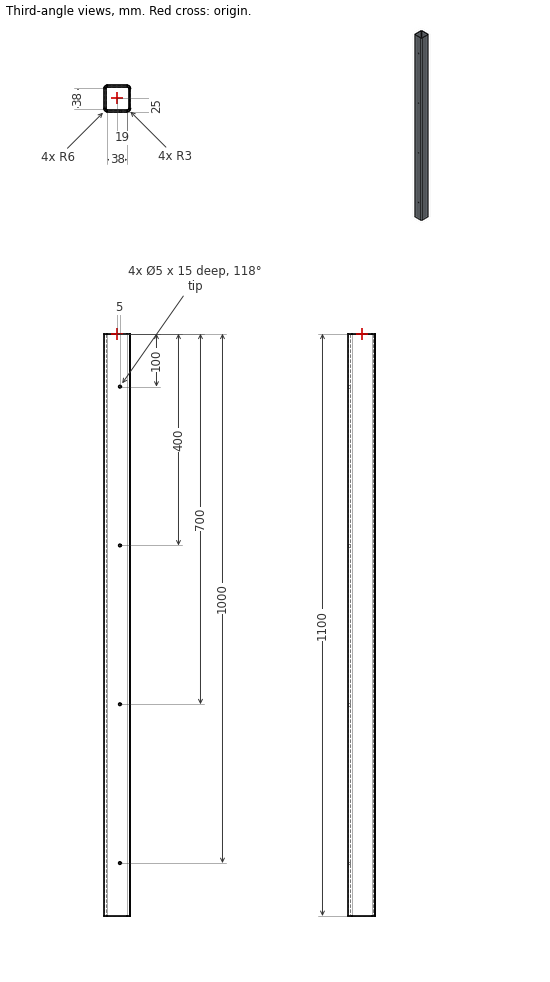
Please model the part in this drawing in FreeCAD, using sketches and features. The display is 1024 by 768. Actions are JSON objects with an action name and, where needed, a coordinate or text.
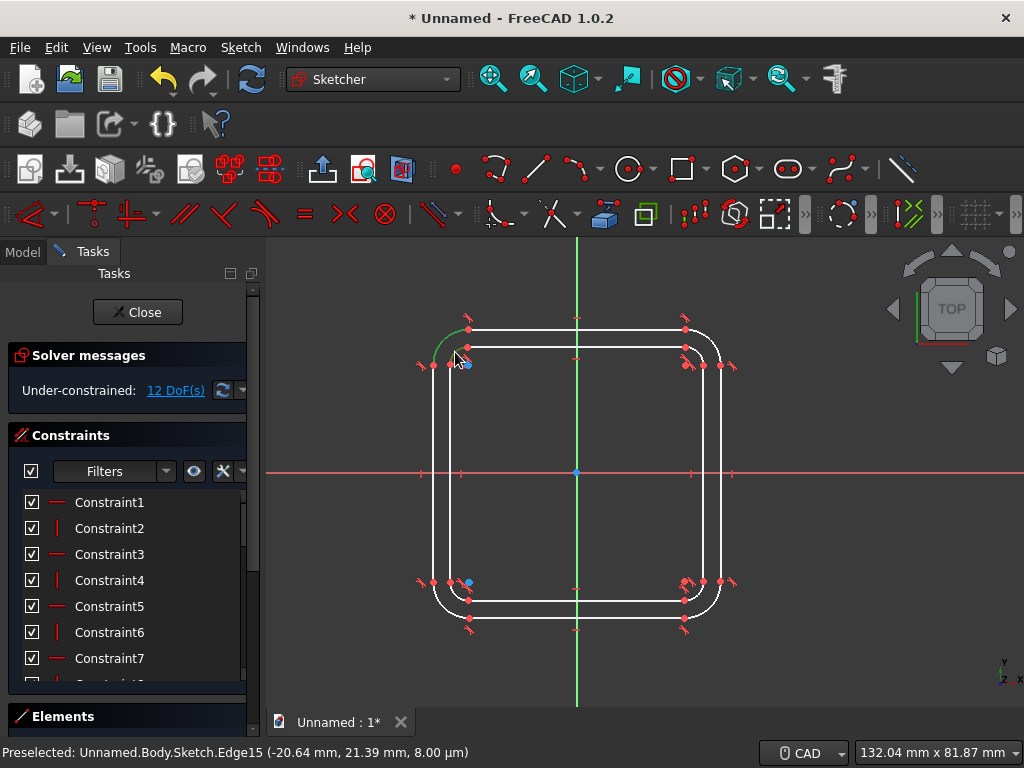
{"action": "left_click", "coordinate": [92, 214]}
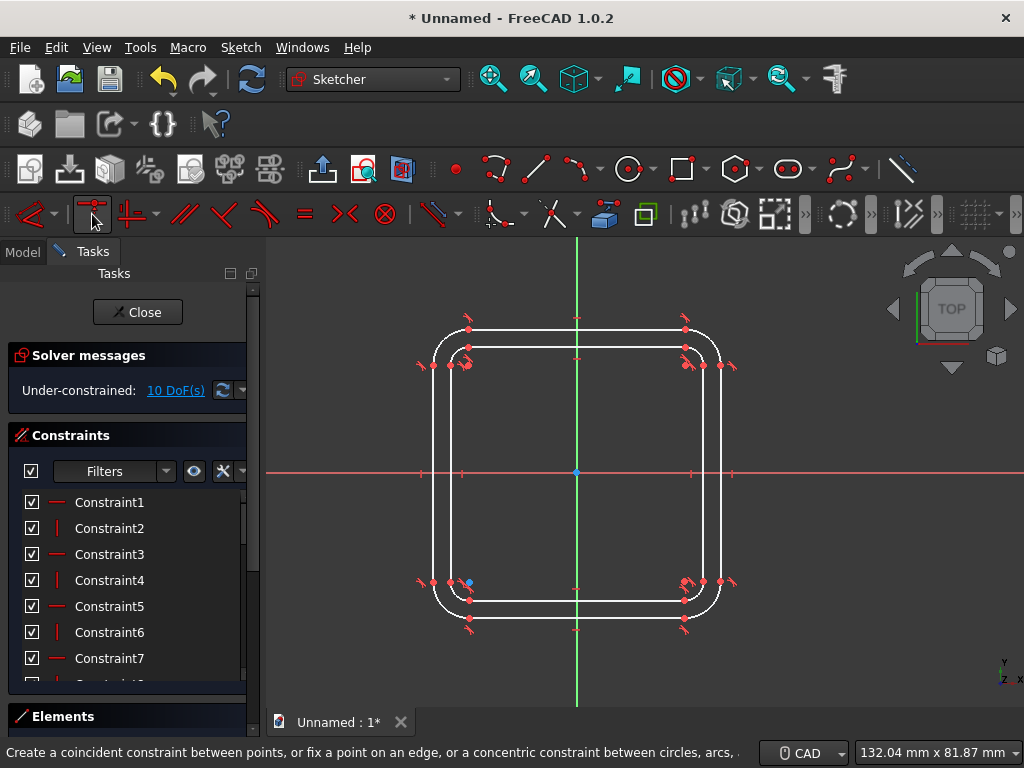
{"action": "left_click", "coordinate": [437, 599]}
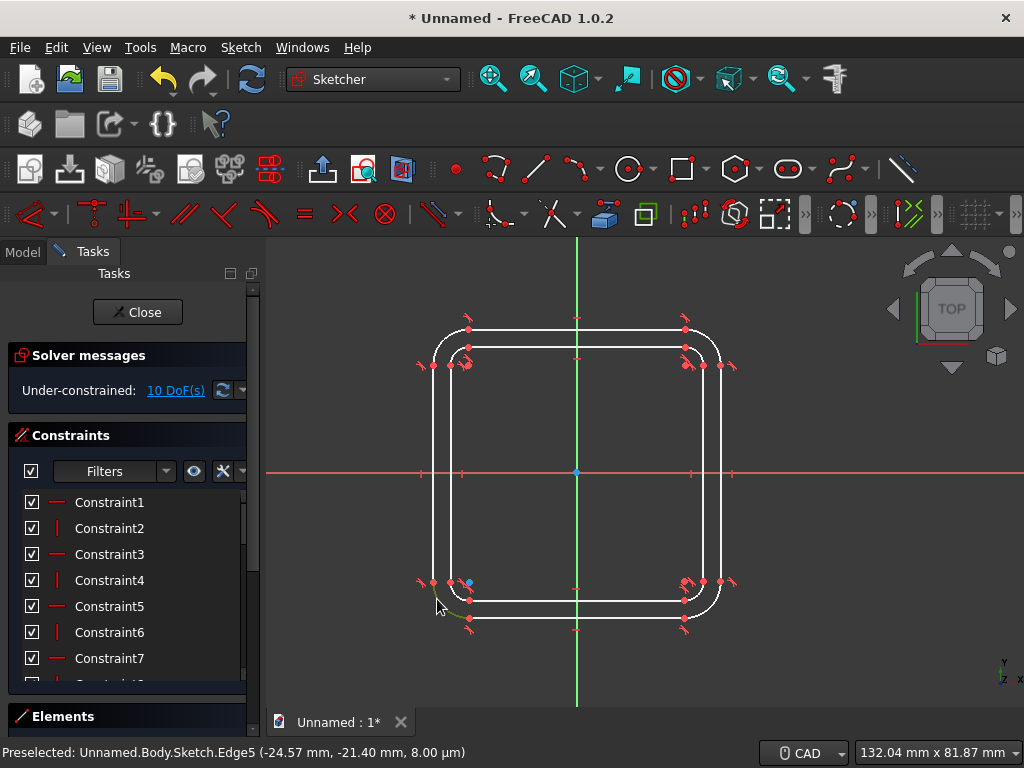
{"action": "left_click", "coordinate": [453, 334]}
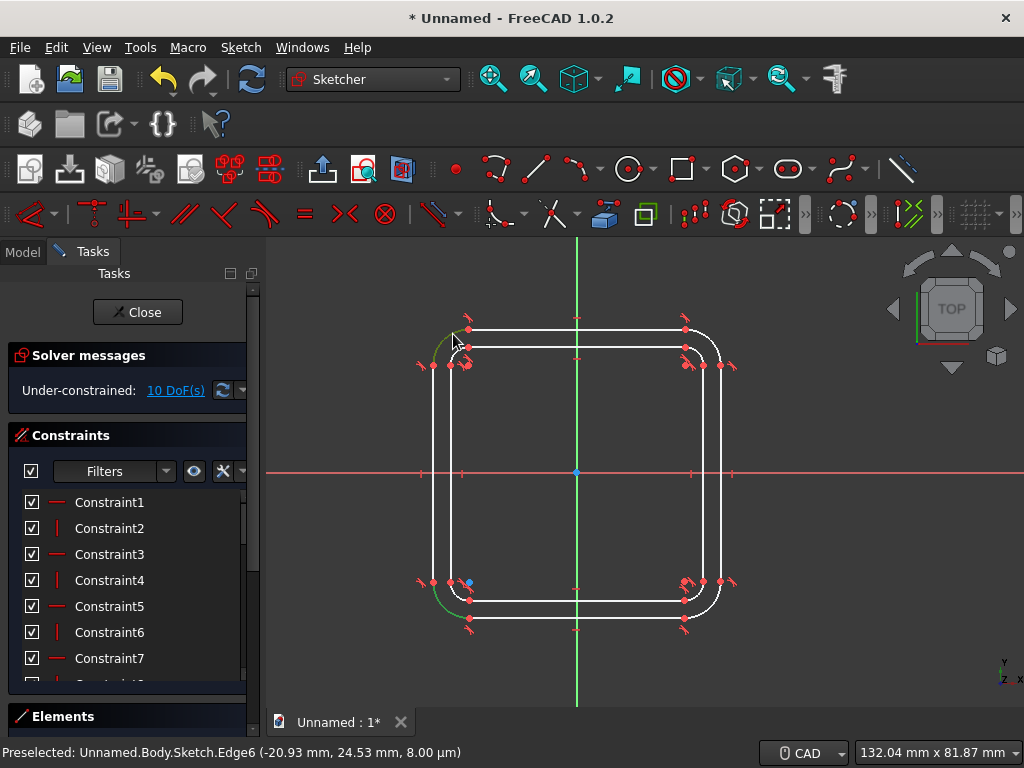
{"action": "left_click", "coordinate": [717, 349]}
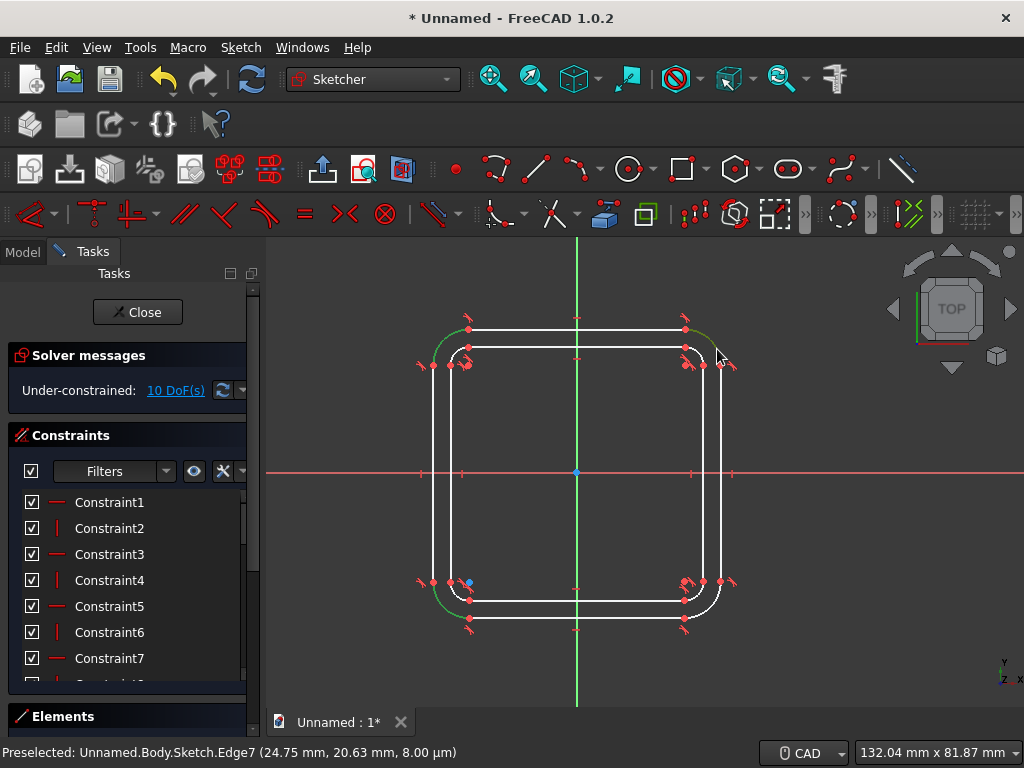
{"action": "left_click", "coordinate": [701, 614]}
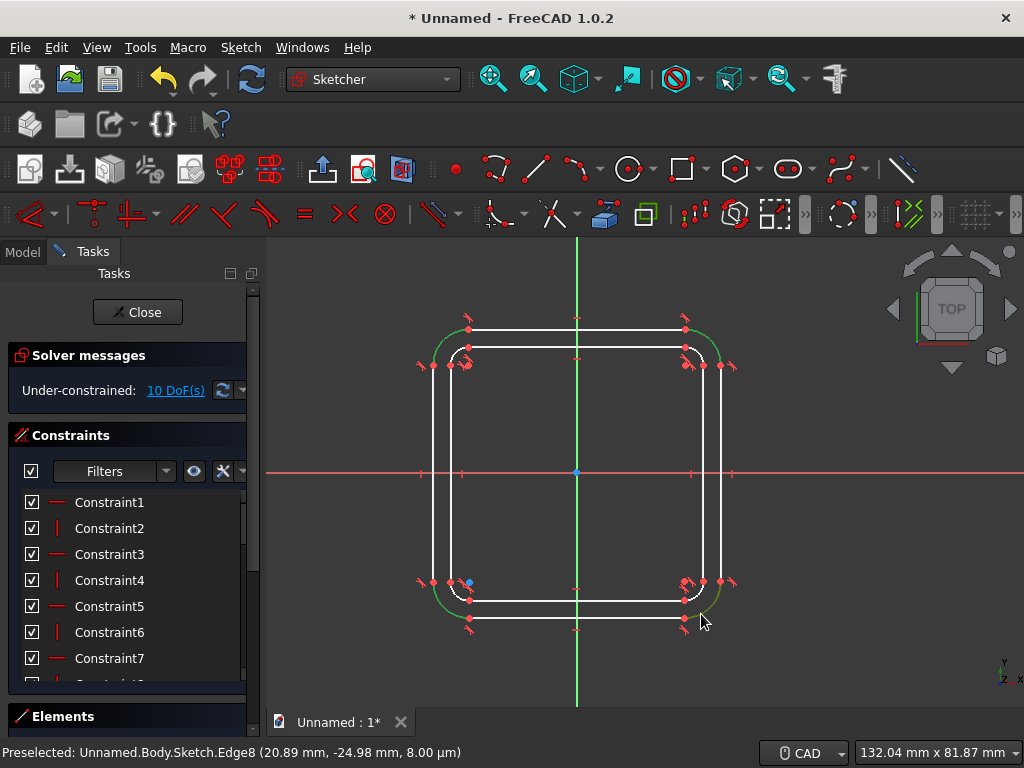
{"action": "key", "text": "e"}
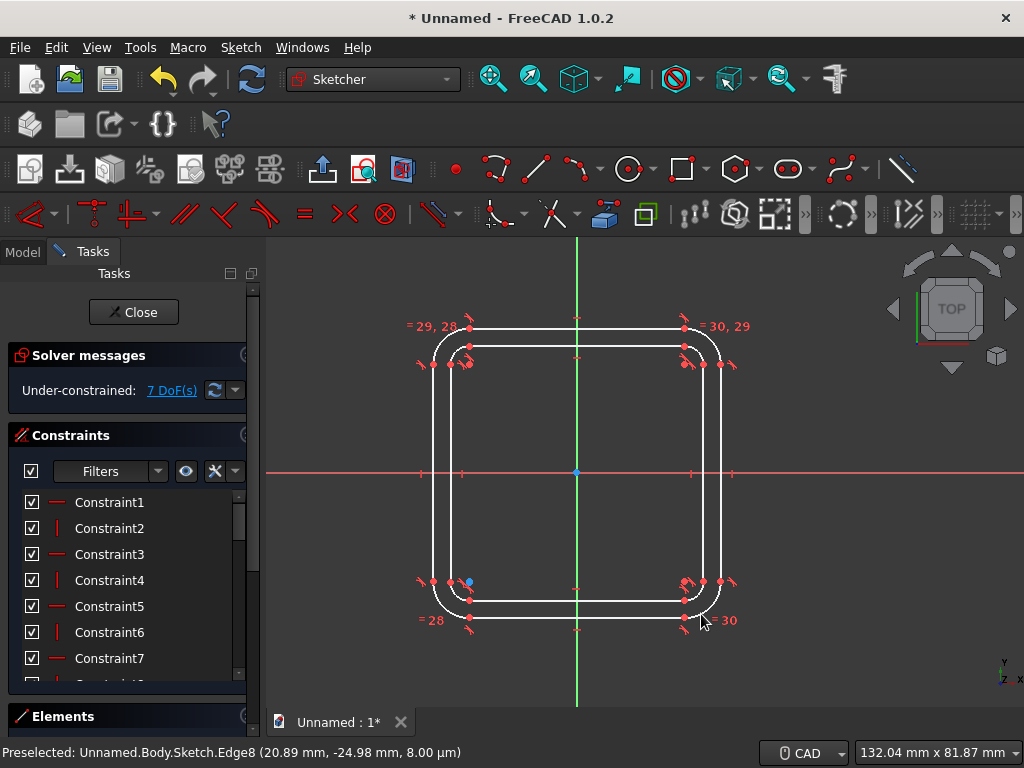
{"action": "left_click", "coordinate": [698, 595]}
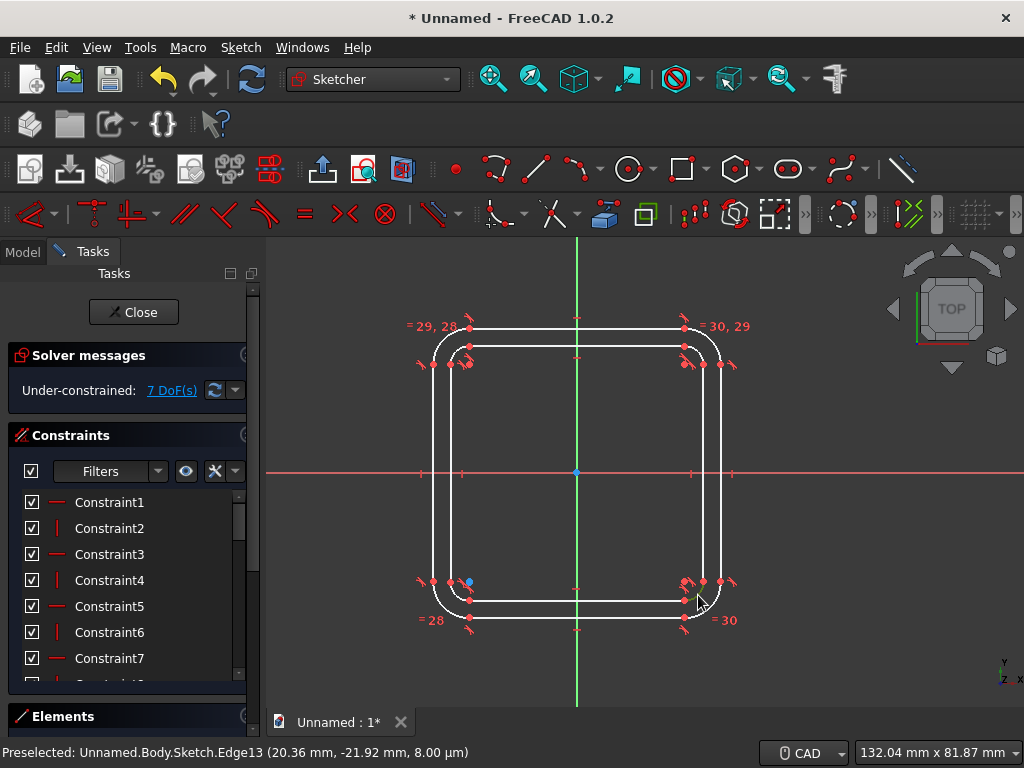
{"action": "left_click", "coordinate": [456, 595]}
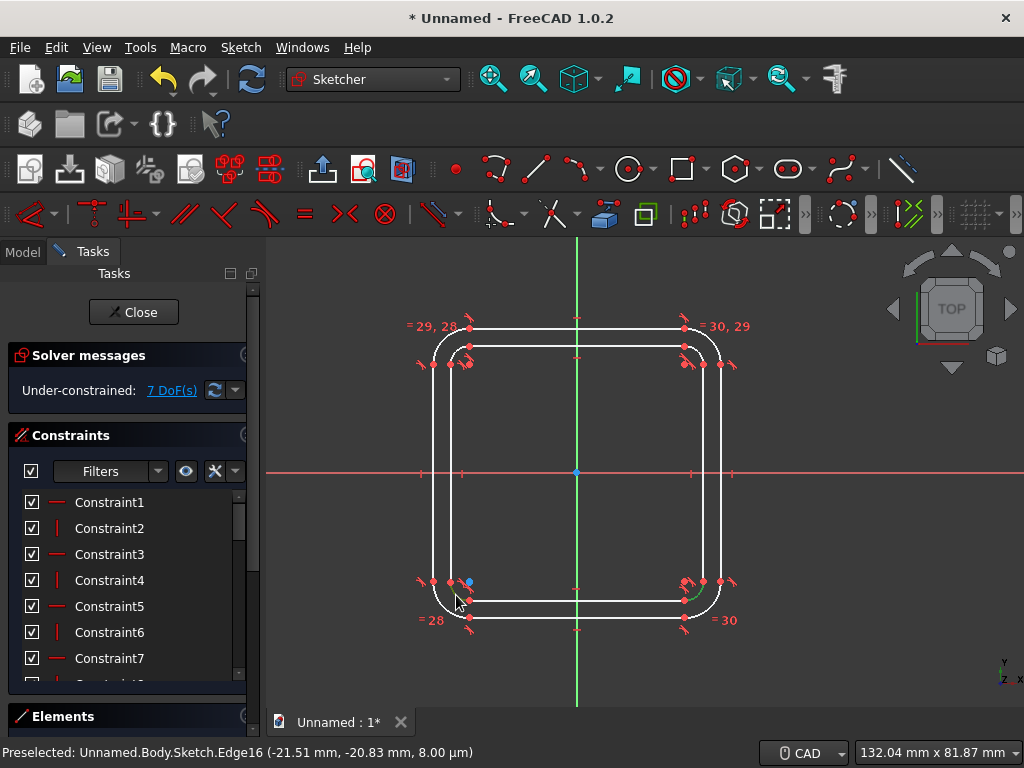
{"action": "left_click", "coordinate": [306, 214]}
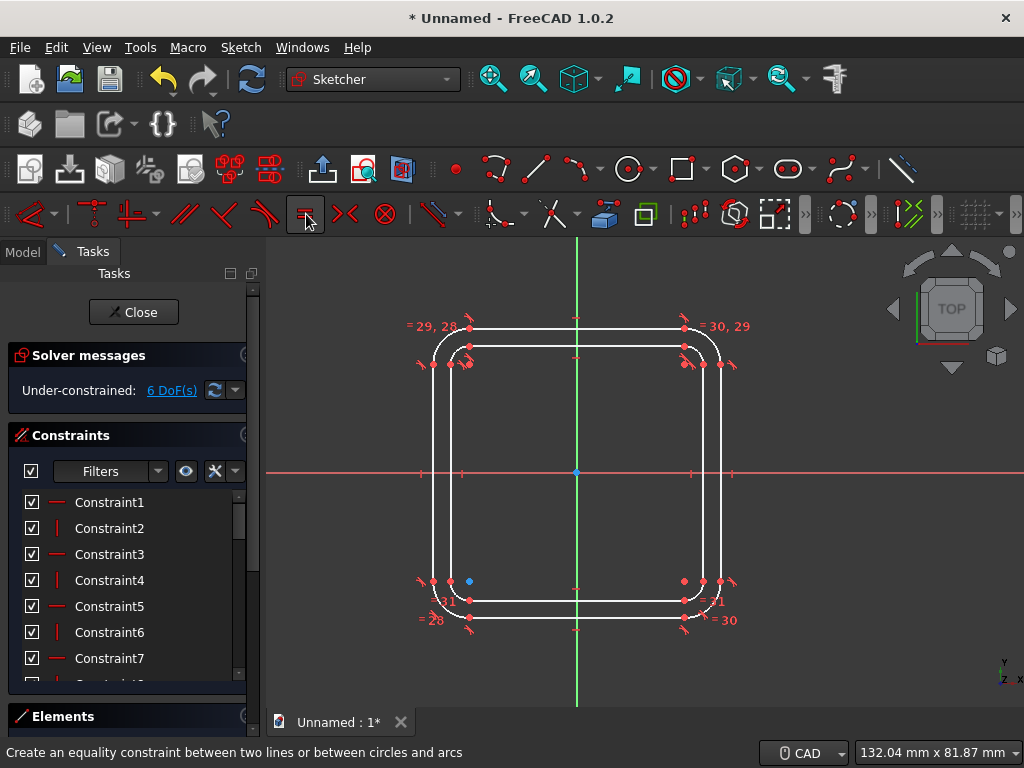
{"action": "left_click", "coordinate": [458, 616]}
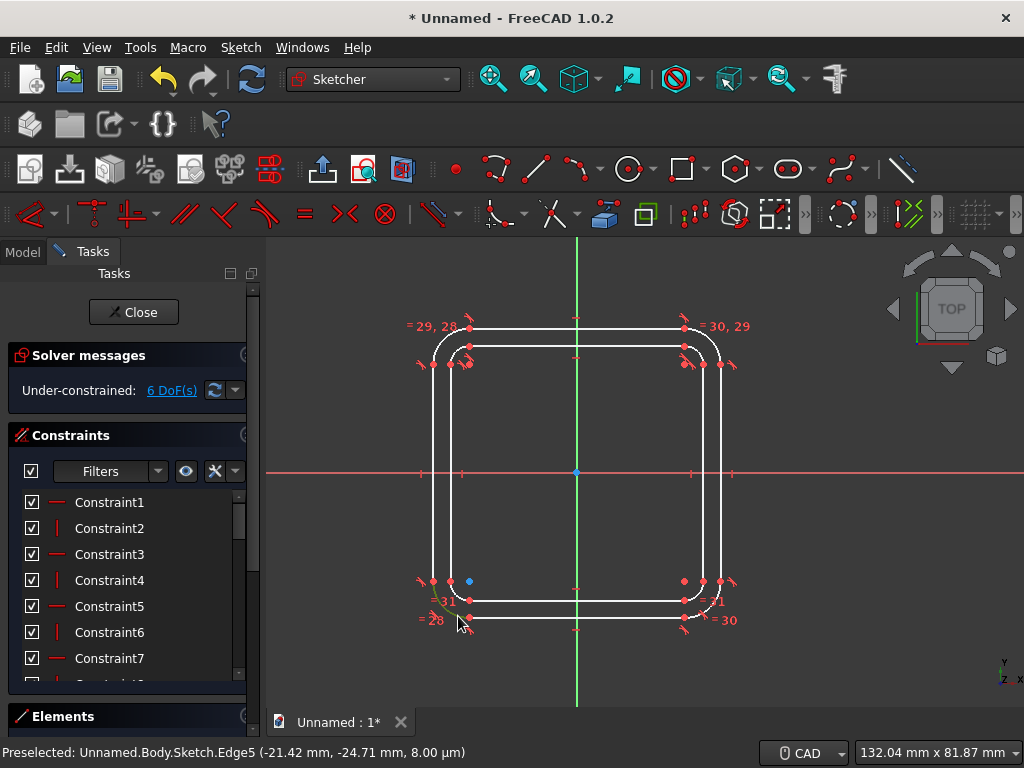
{"action": "key", "text": "k r"}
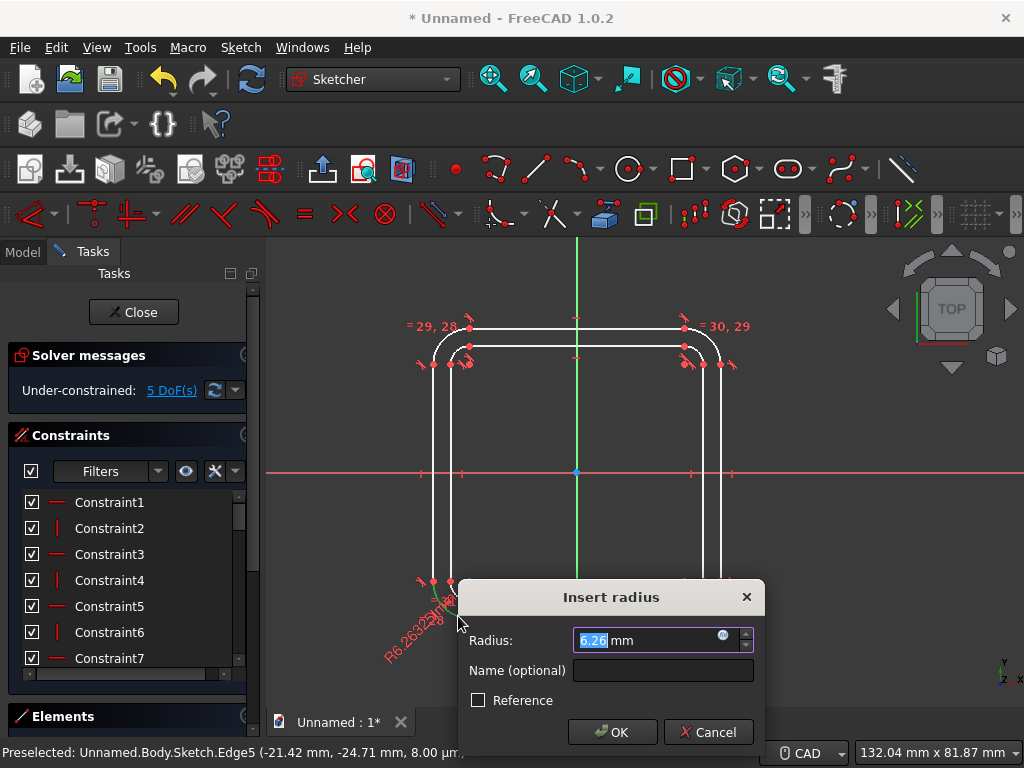
{"action": "type", "text": "6"}
{"action": "key", "text": "Return"}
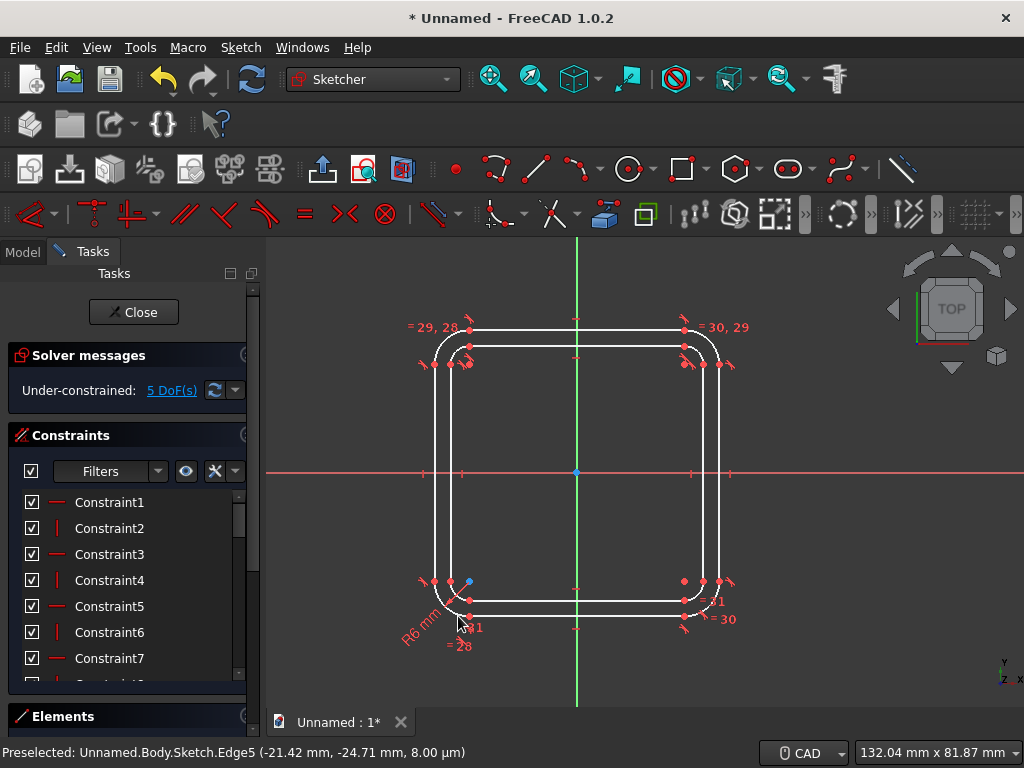
{"action": "scroll", "coordinate": [698, 595], "scroll_direction": "up", "scroll_amount": 5}